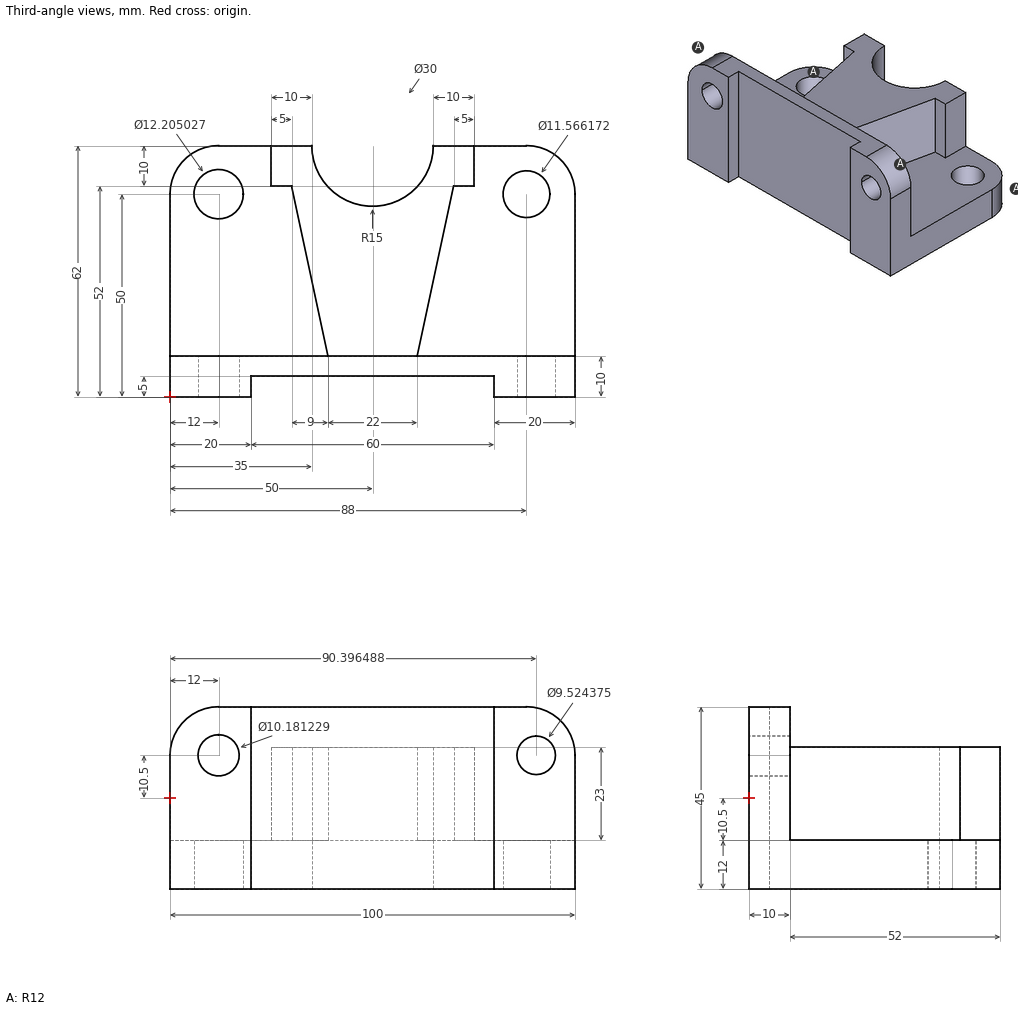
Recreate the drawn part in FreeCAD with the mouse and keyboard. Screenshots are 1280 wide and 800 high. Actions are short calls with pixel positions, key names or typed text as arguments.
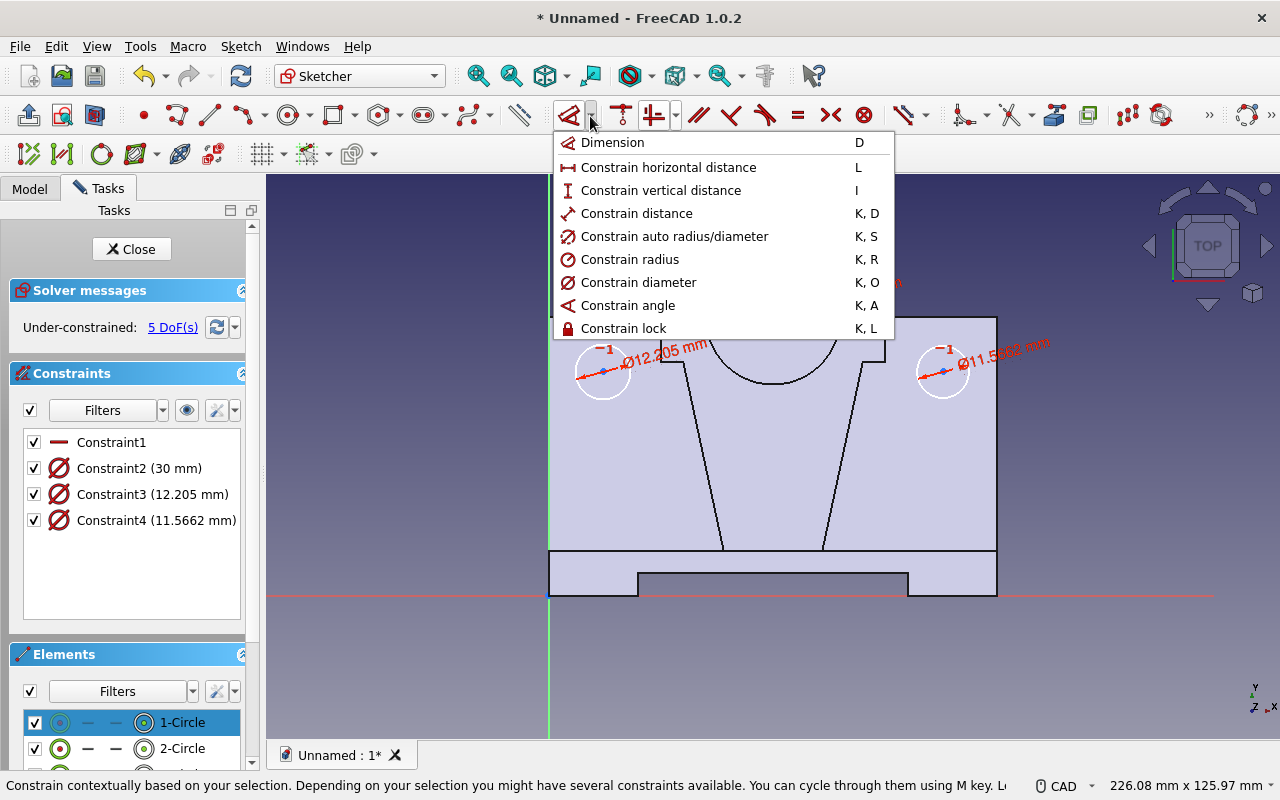
click(724, 168)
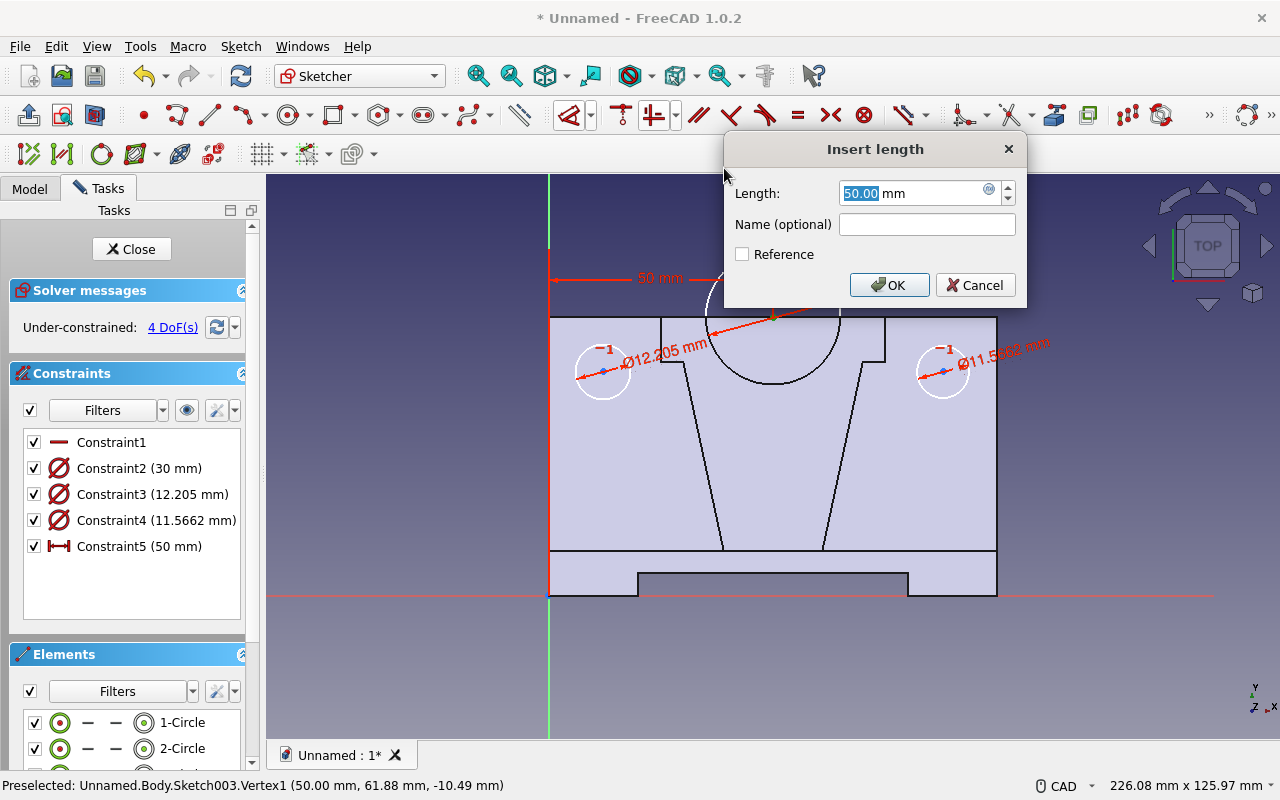
text(50)
key(Return)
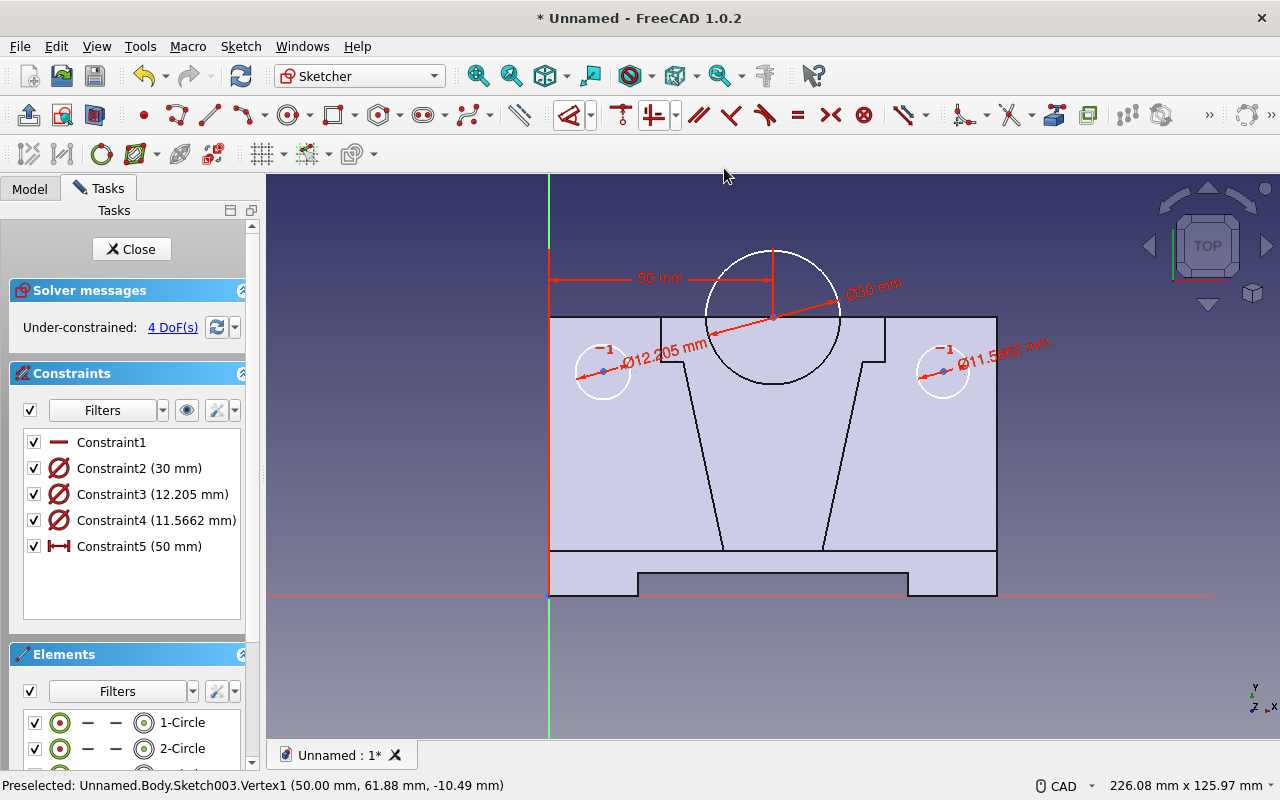
click(773, 318)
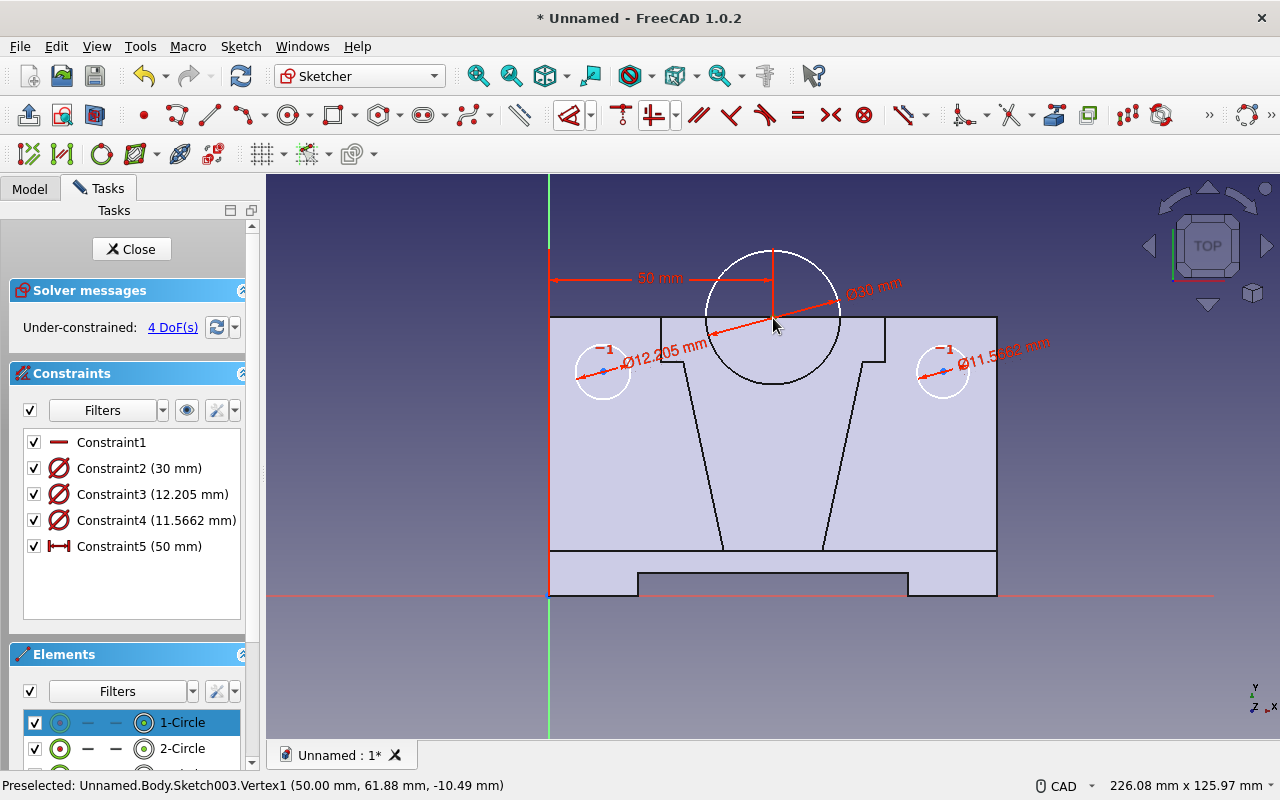
key(i)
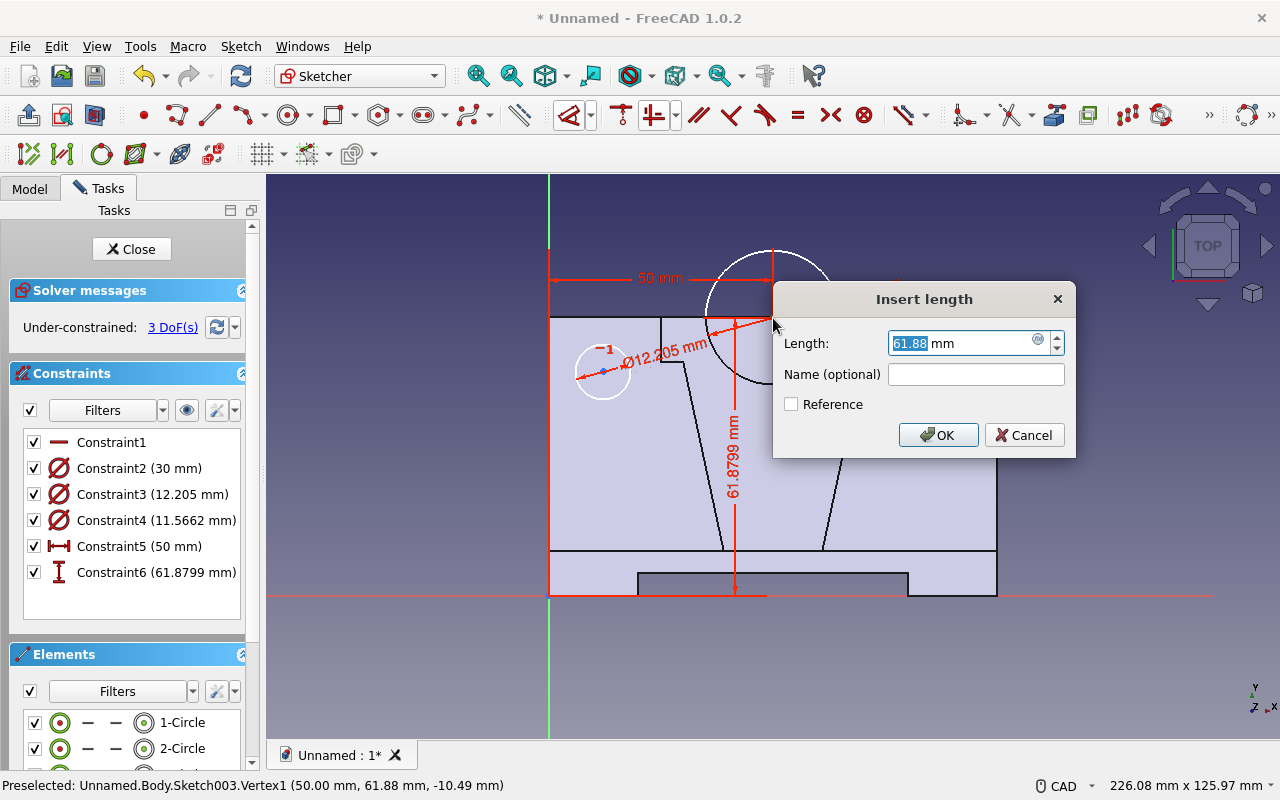
text(62)
key(Return)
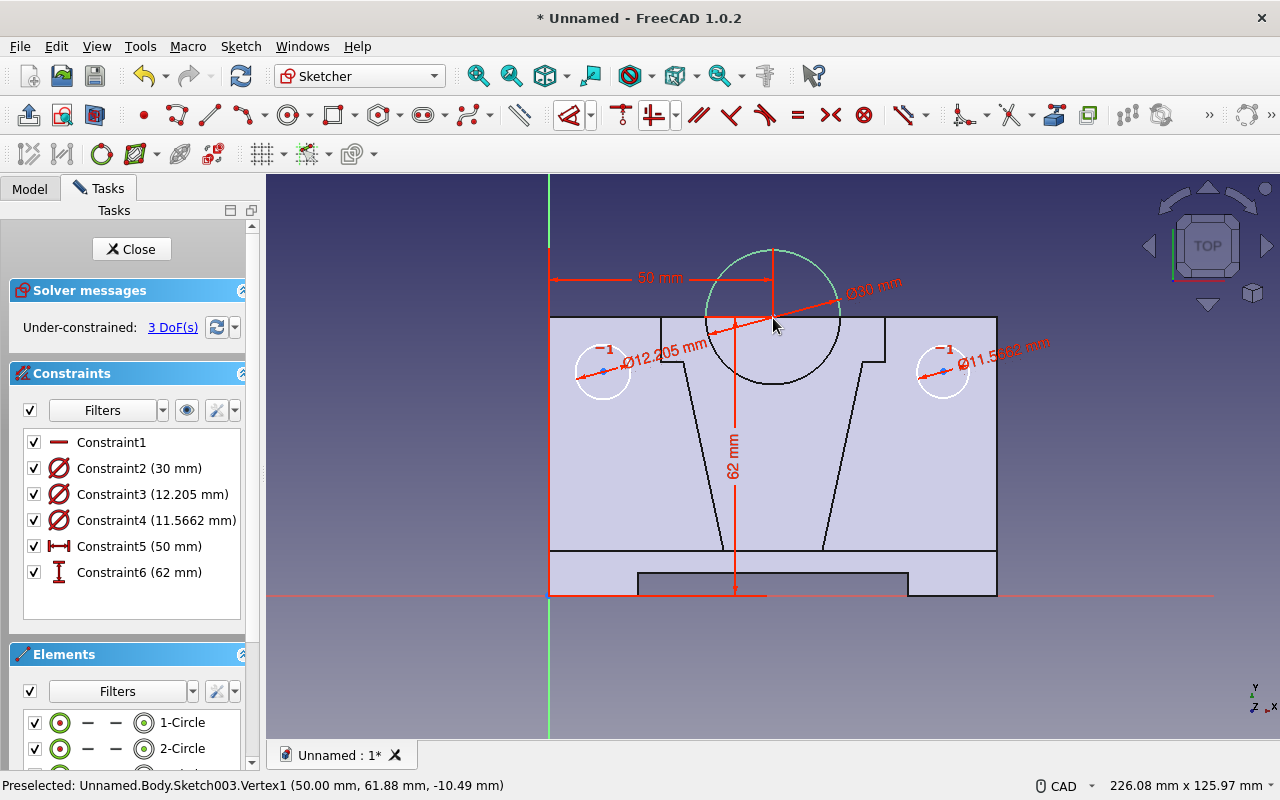
click(603, 372)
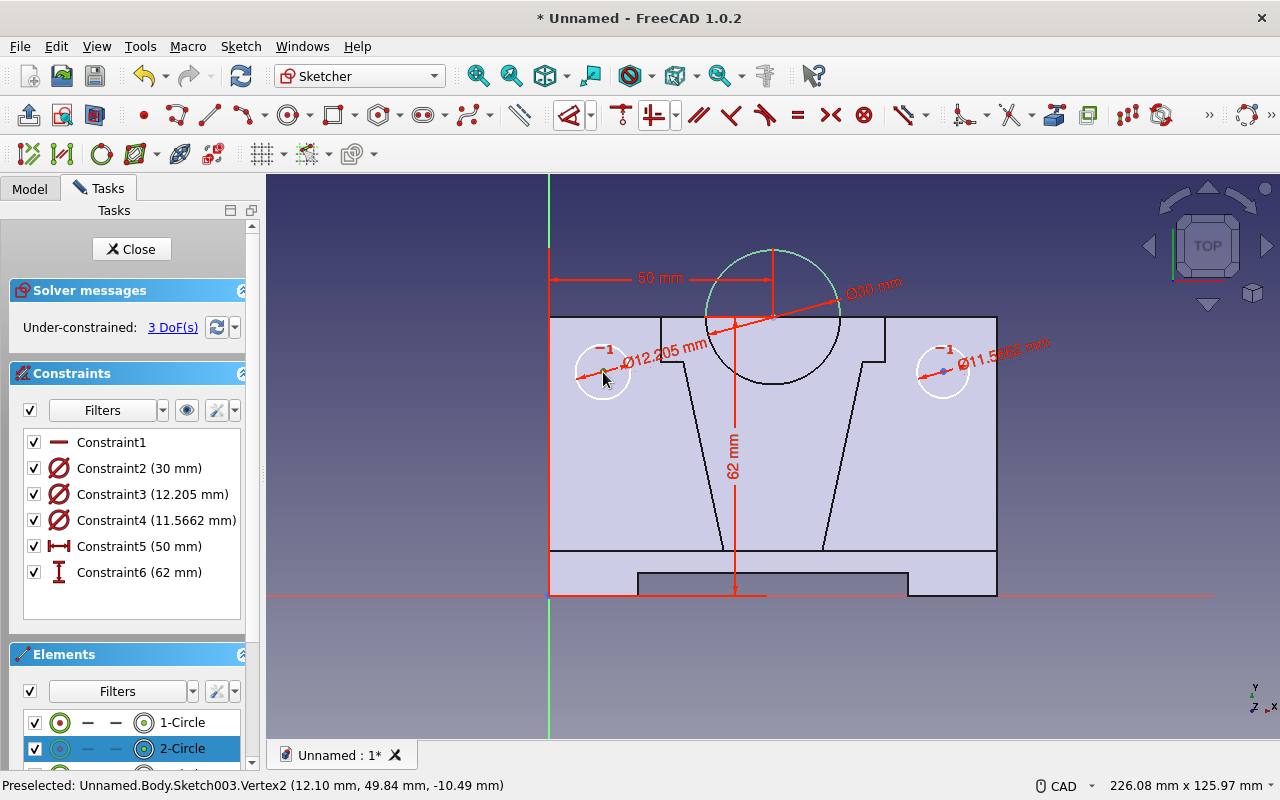
key(l)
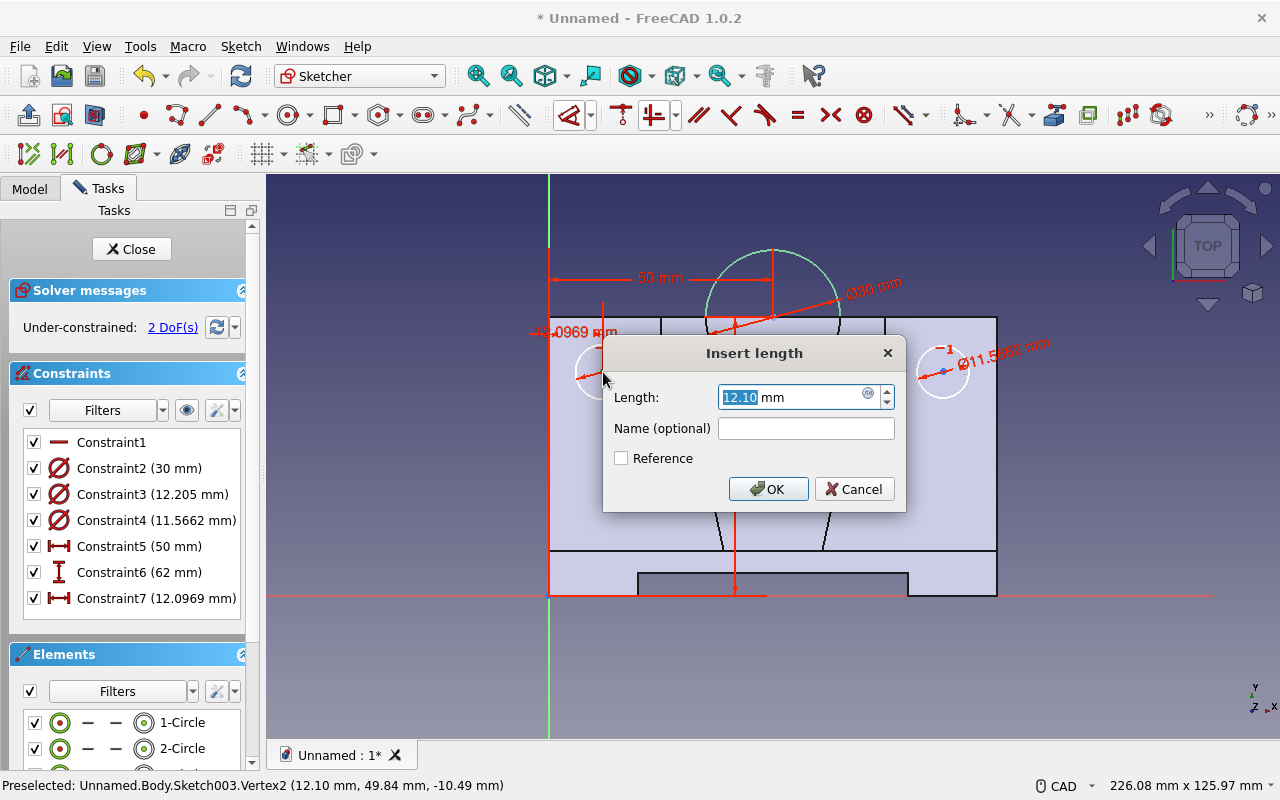
text(12)
key(Return)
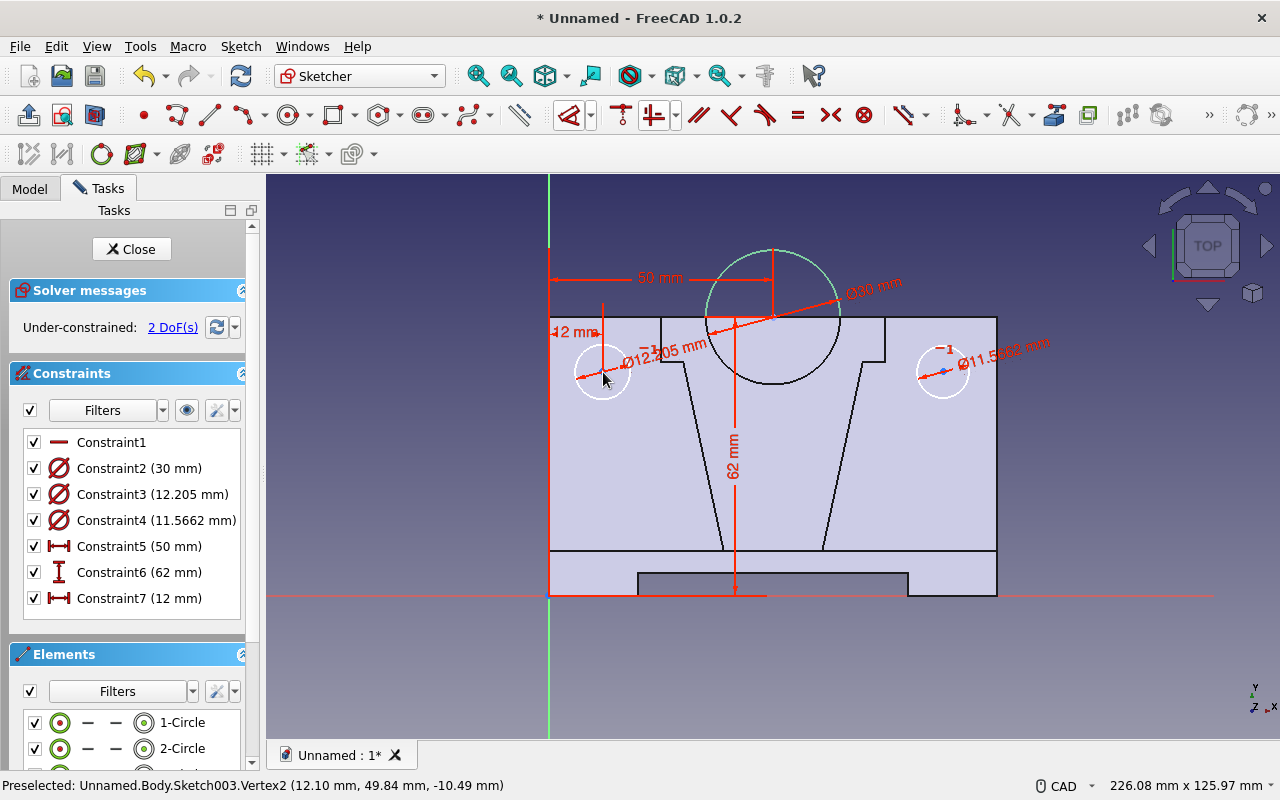
click(603, 372)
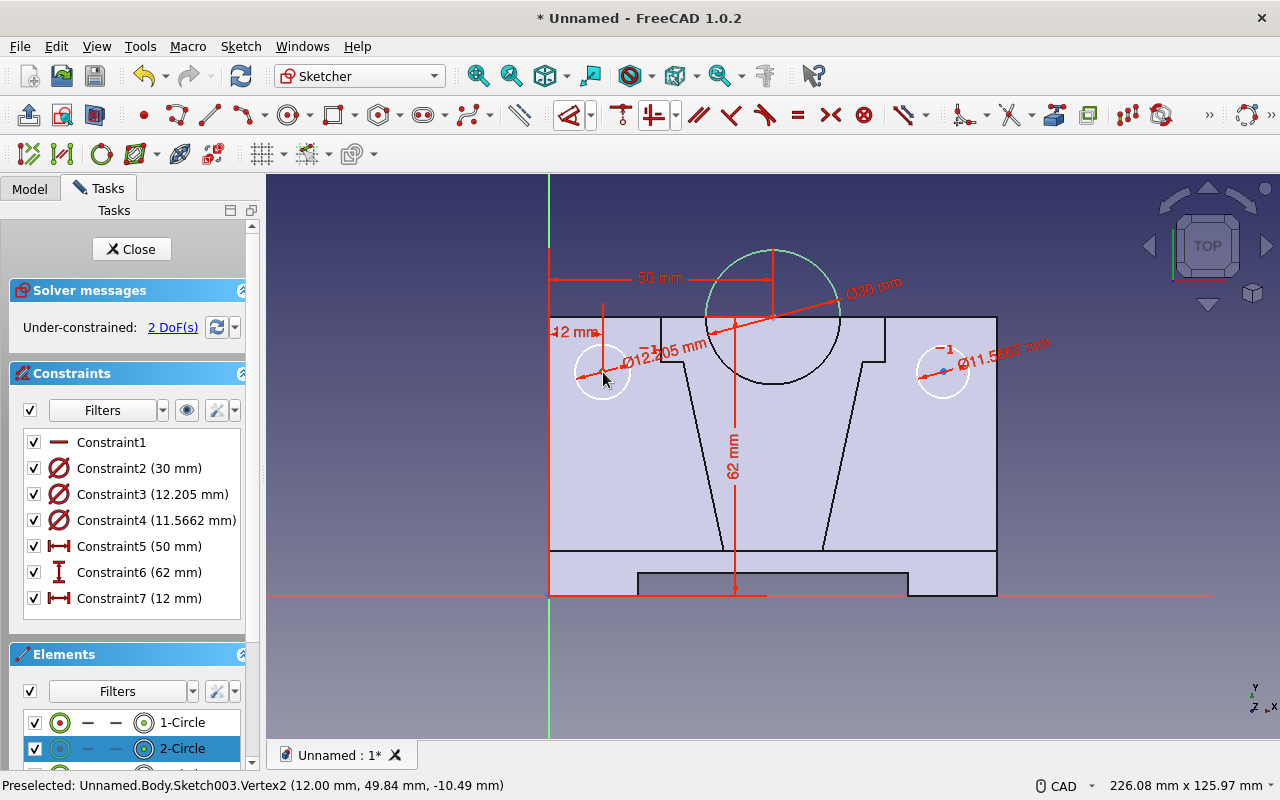
key(i)